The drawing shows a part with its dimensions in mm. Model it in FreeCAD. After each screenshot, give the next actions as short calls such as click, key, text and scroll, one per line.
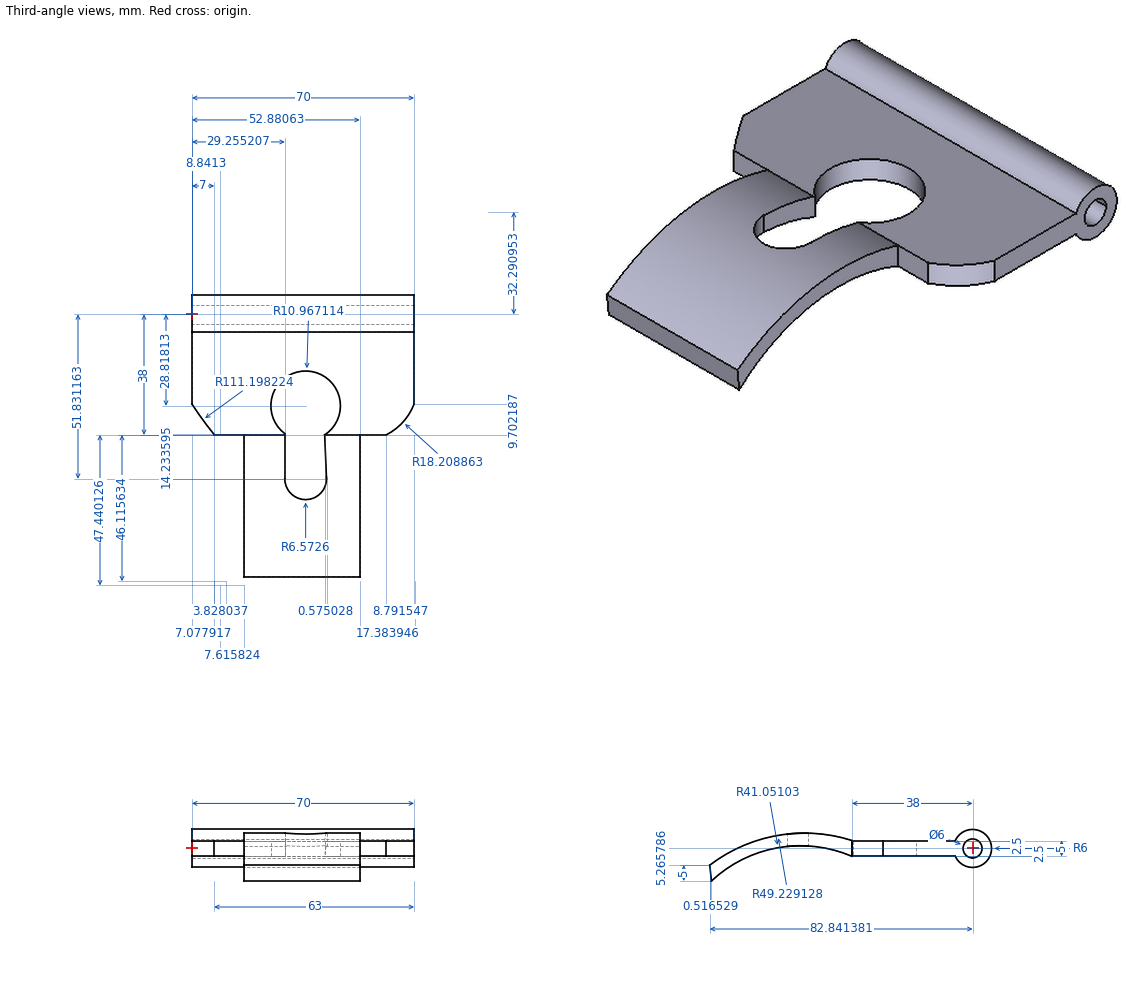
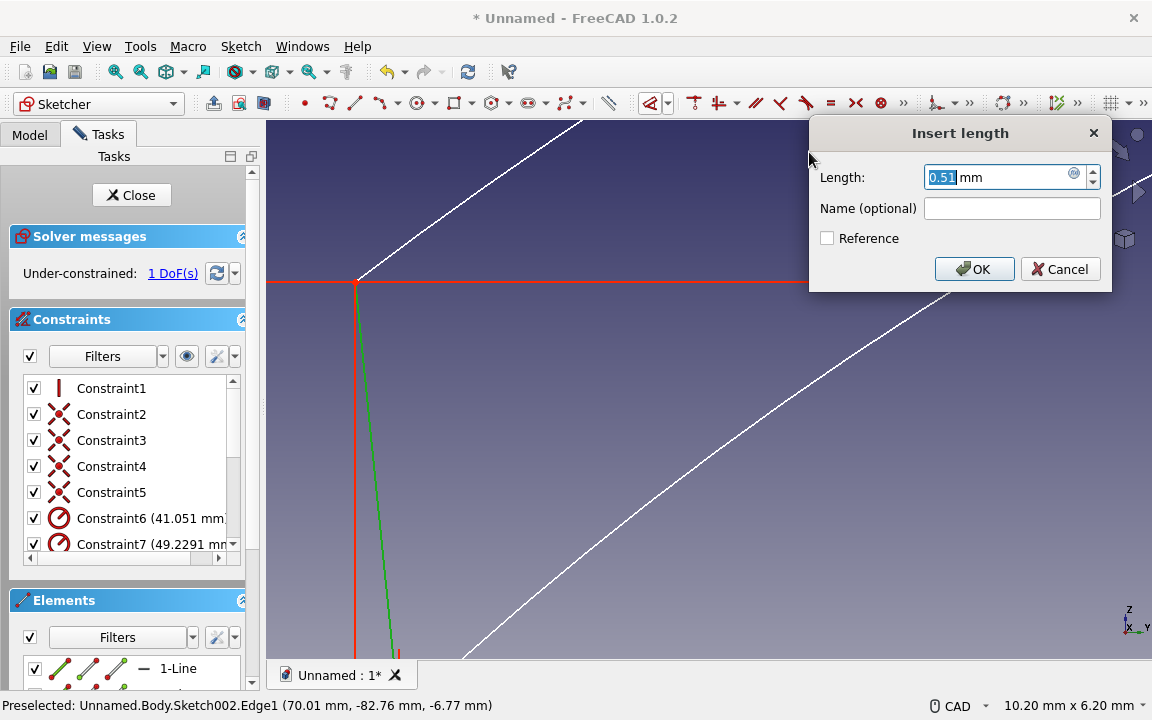
text(0.516529)
key(Return)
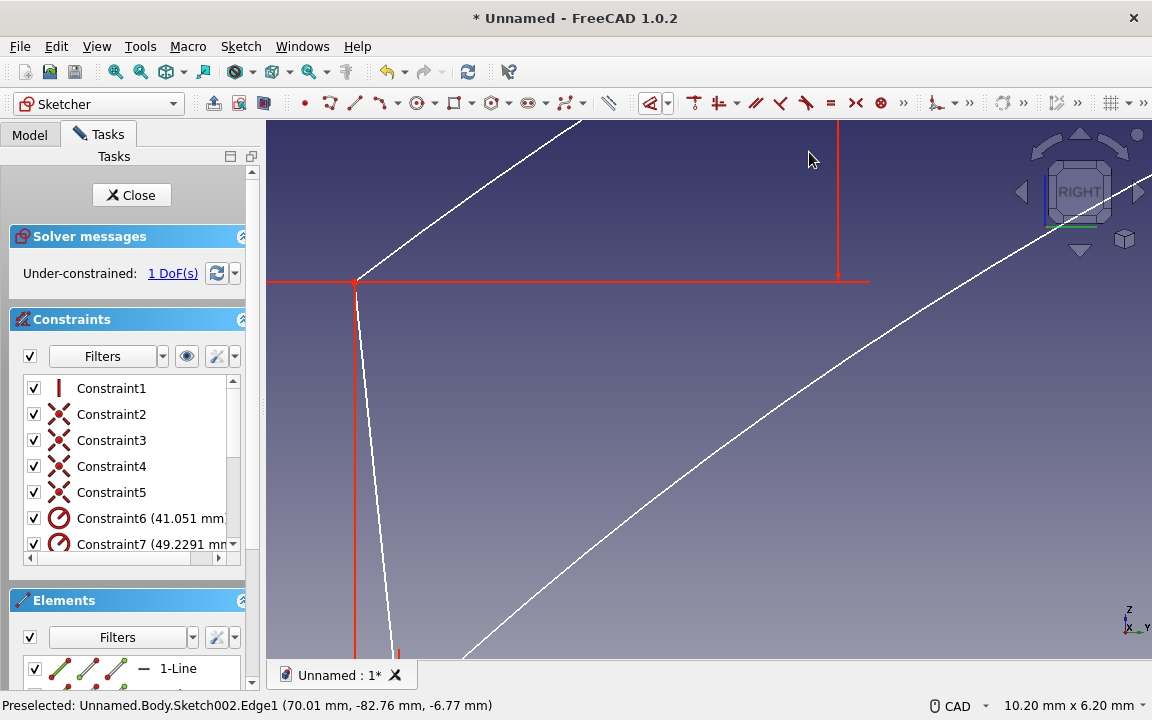
scroll(374, 413, down, 13)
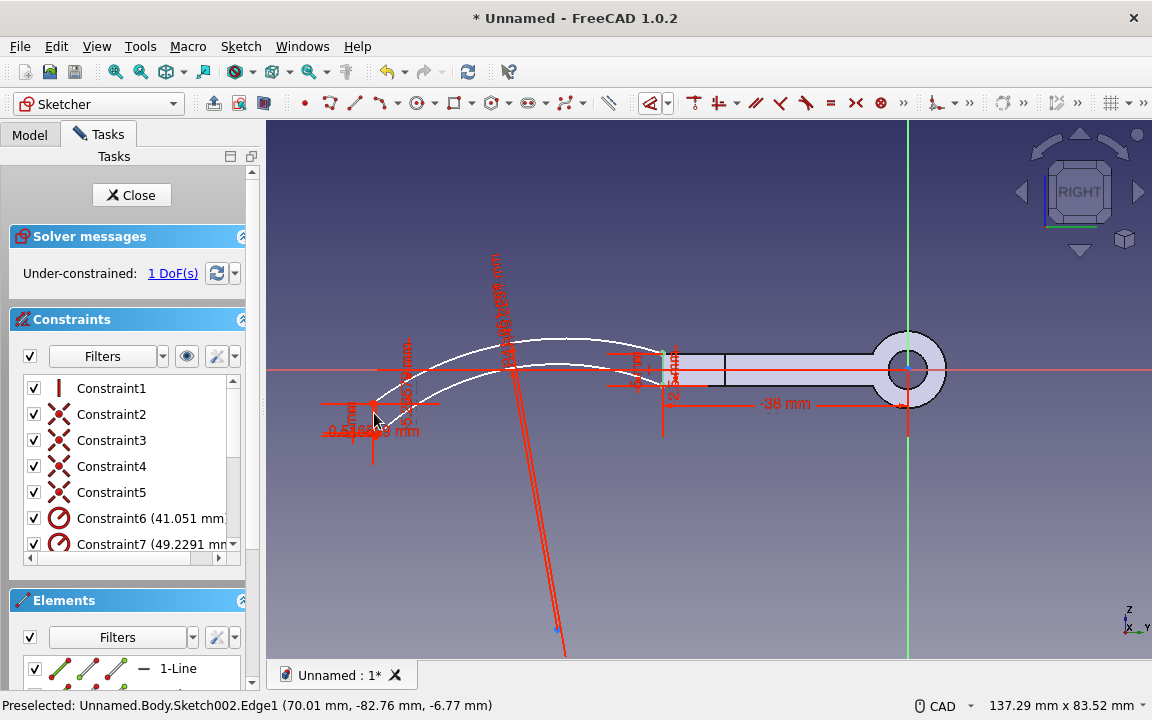
click(373, 404)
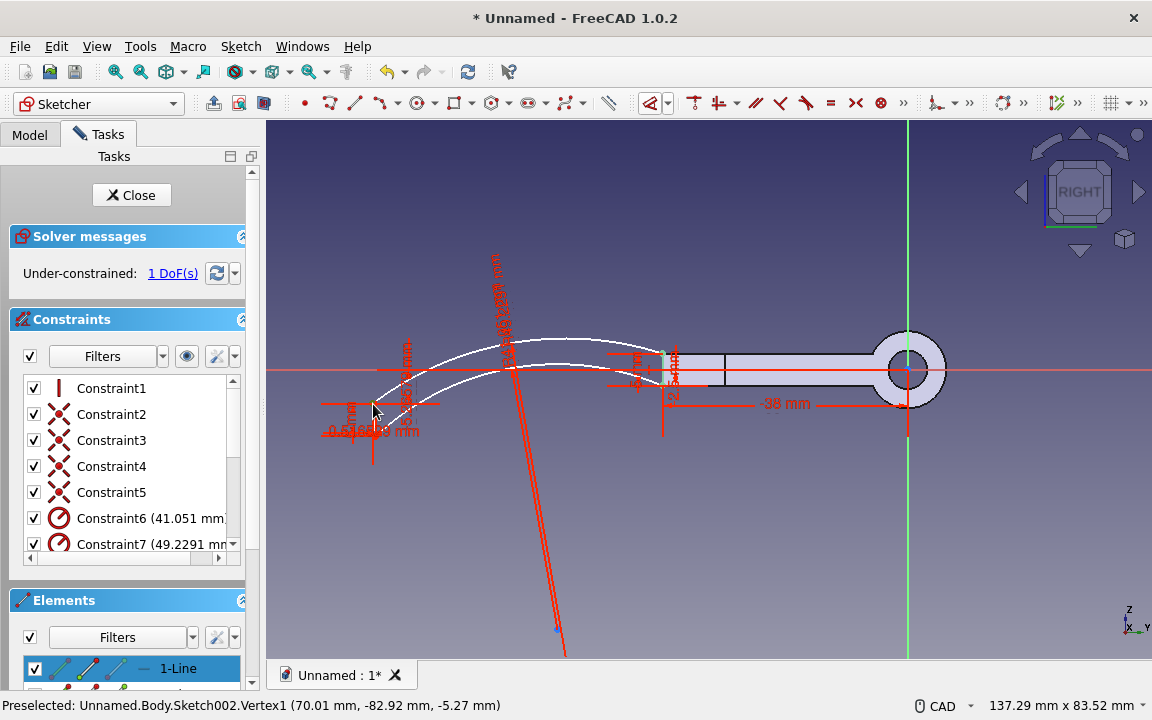
key(l)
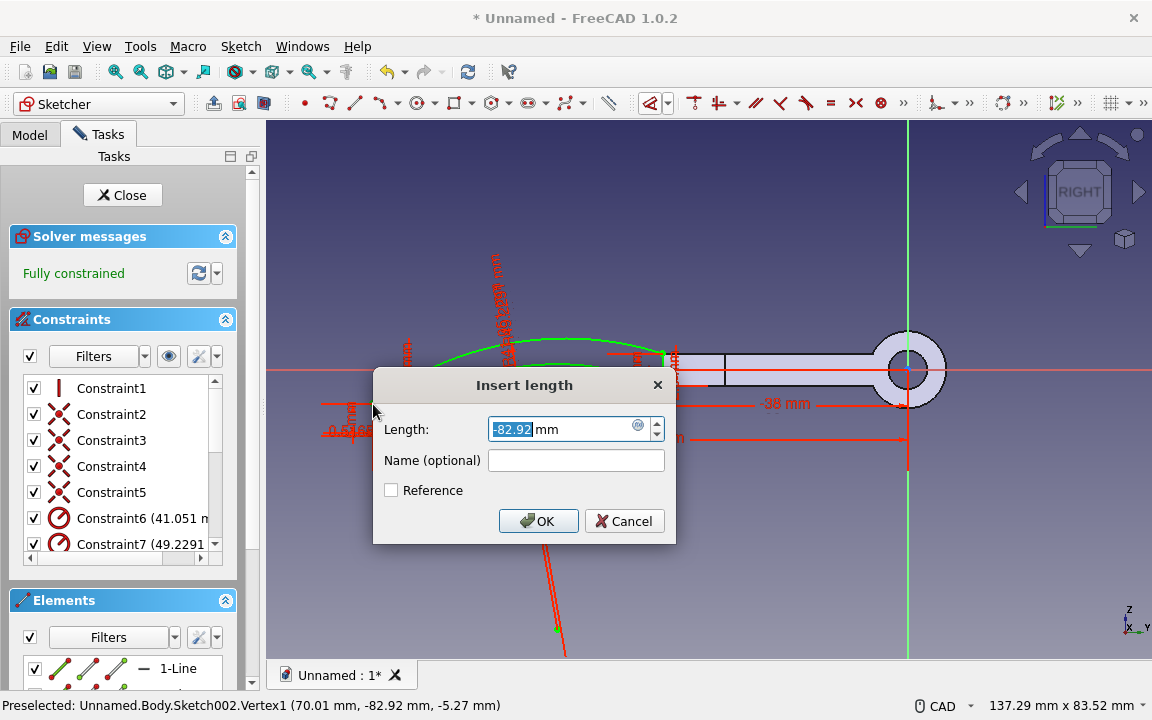
text(-82.841381)
key(Return)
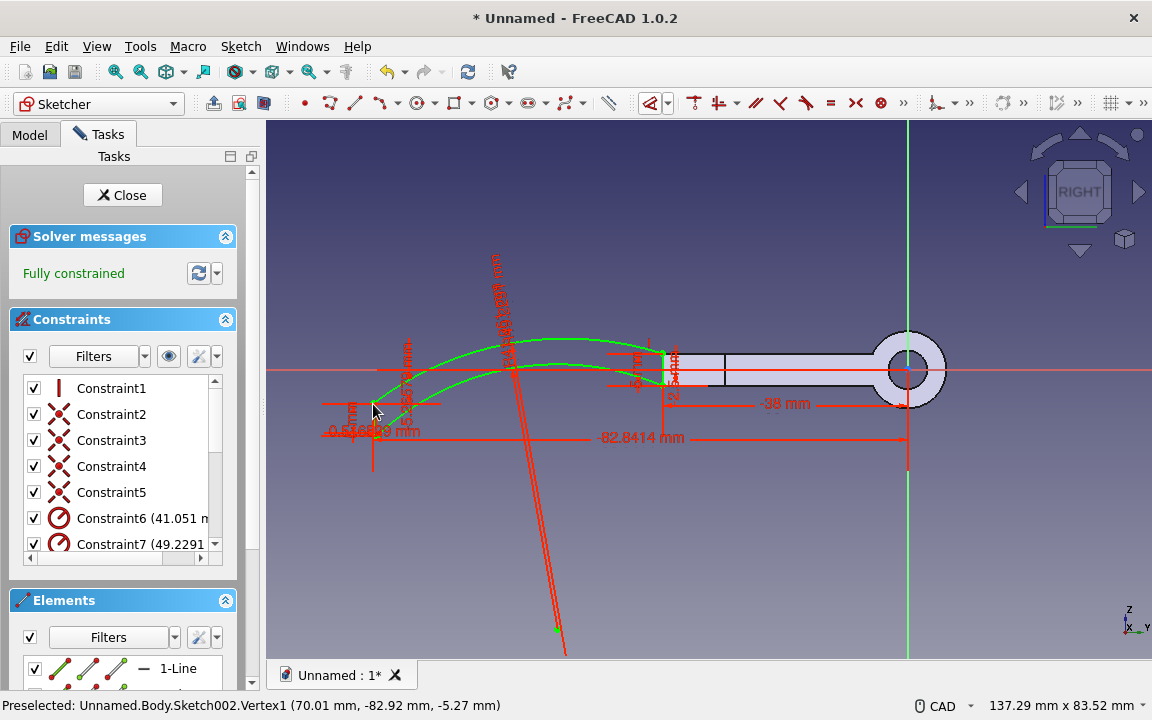
click(123, 195)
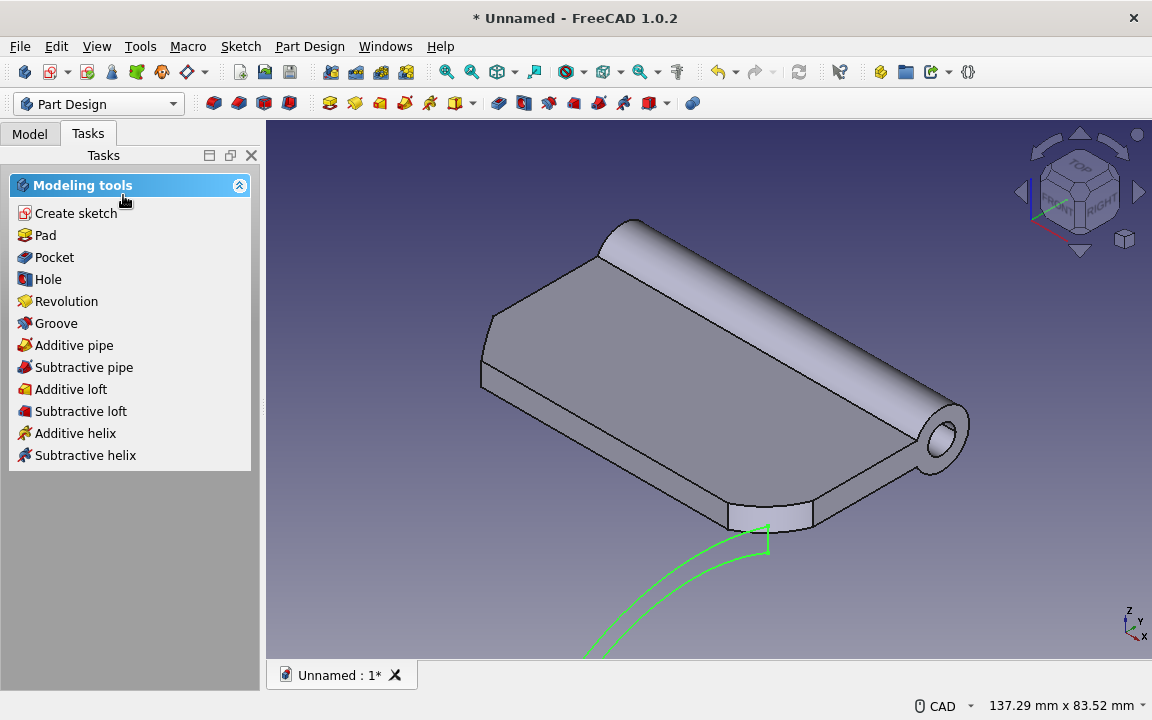
click(330, 104)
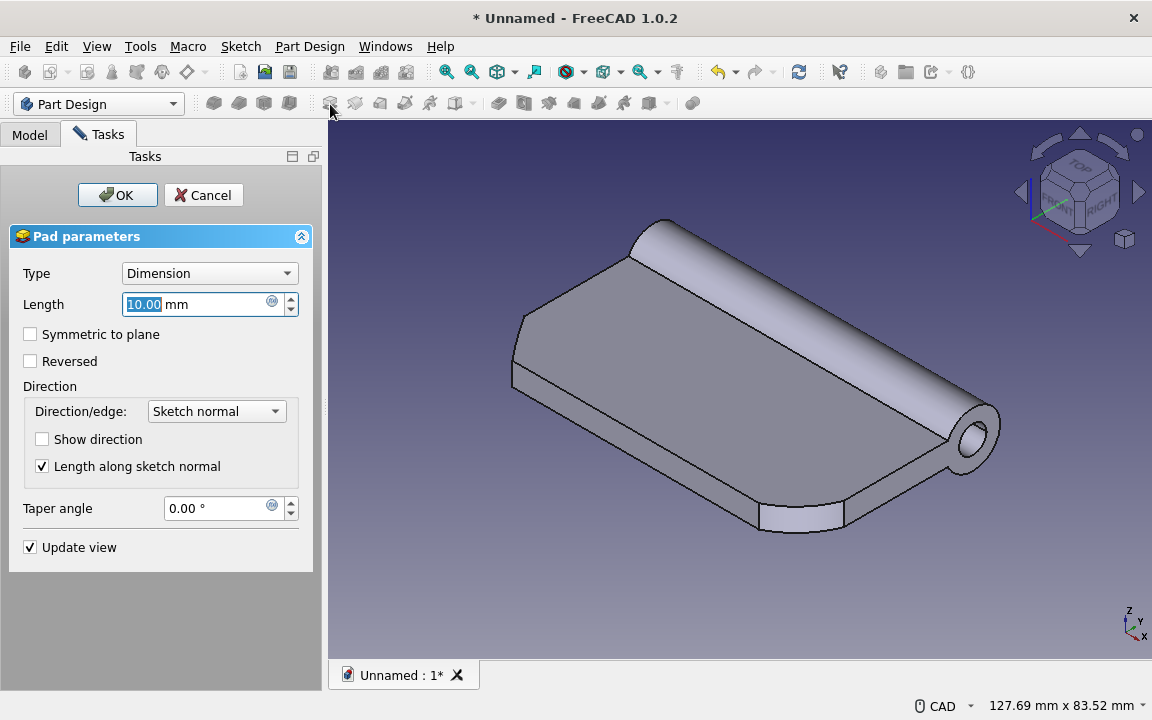
text(63)
key(Tab)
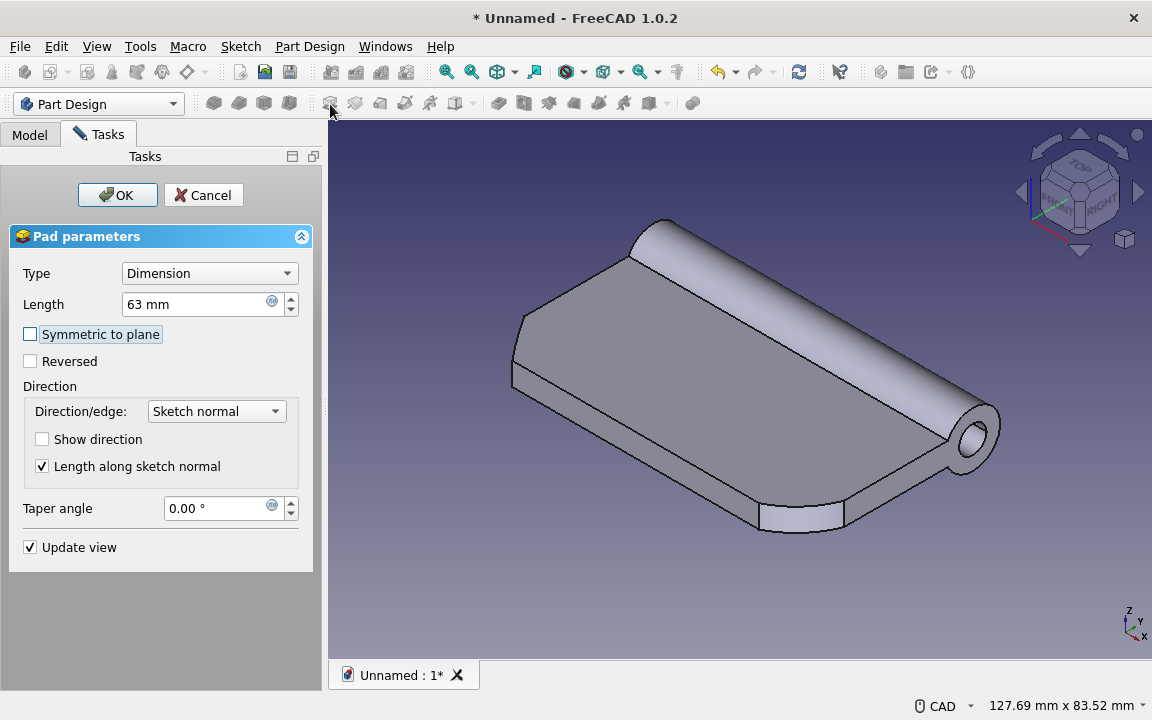
click(31, 361)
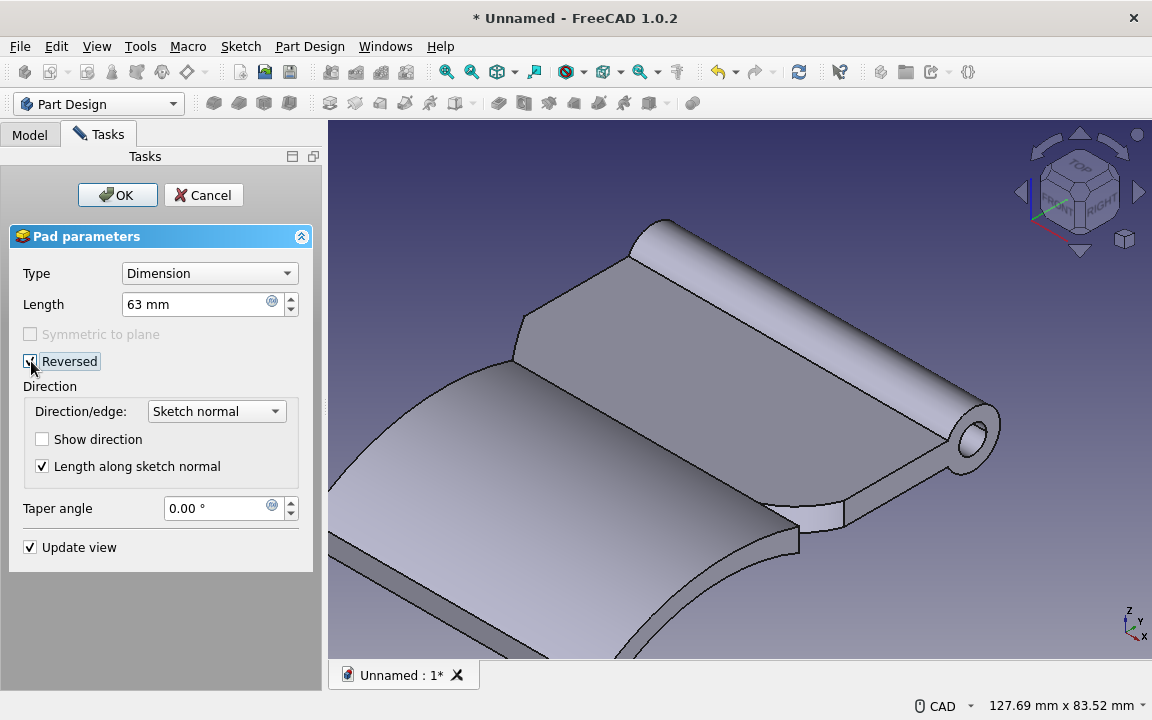
click(118, 195)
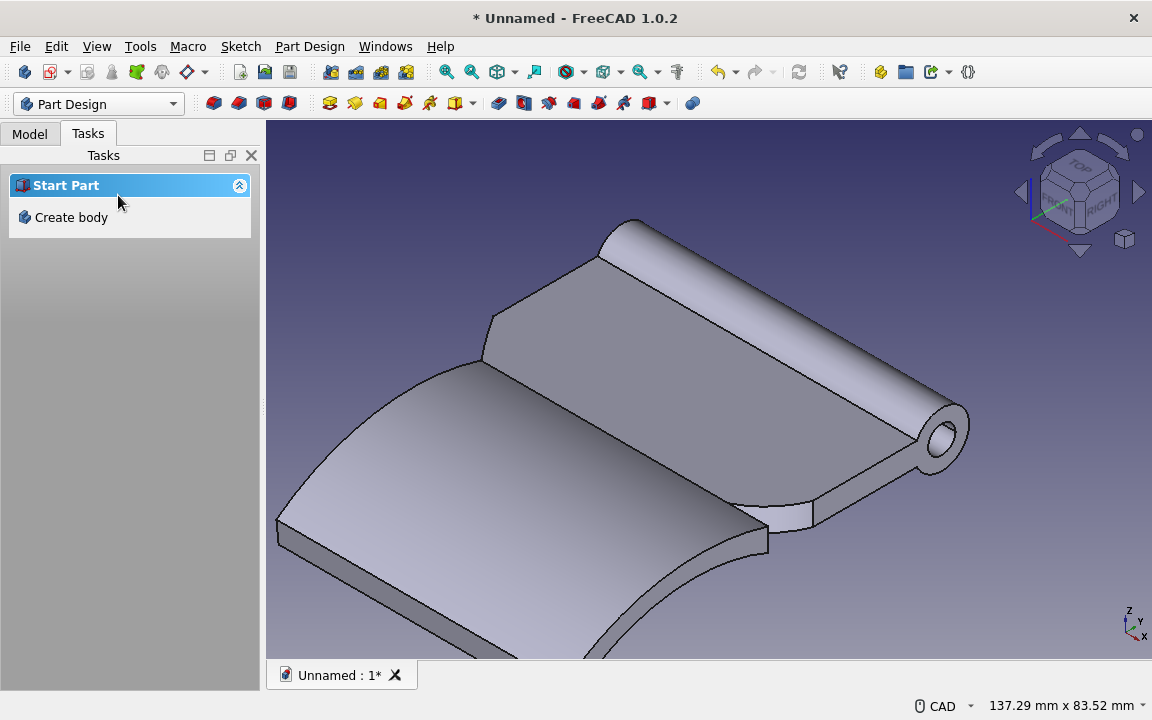
click(447, 72)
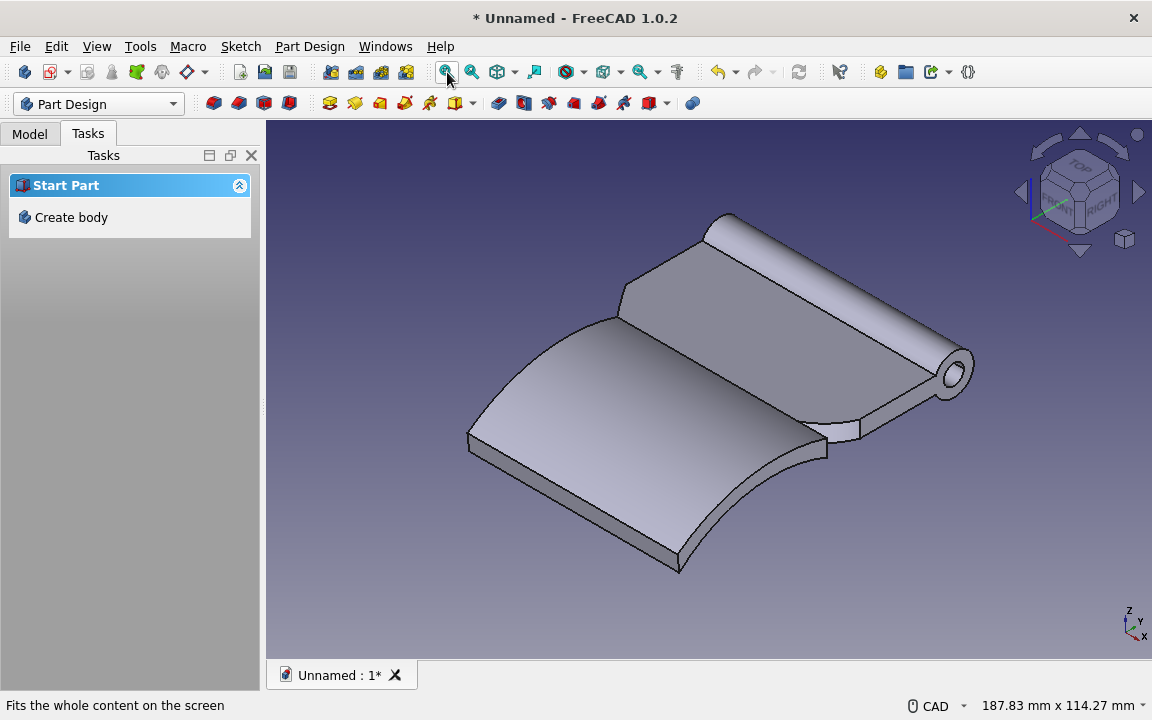
click(50, 72)